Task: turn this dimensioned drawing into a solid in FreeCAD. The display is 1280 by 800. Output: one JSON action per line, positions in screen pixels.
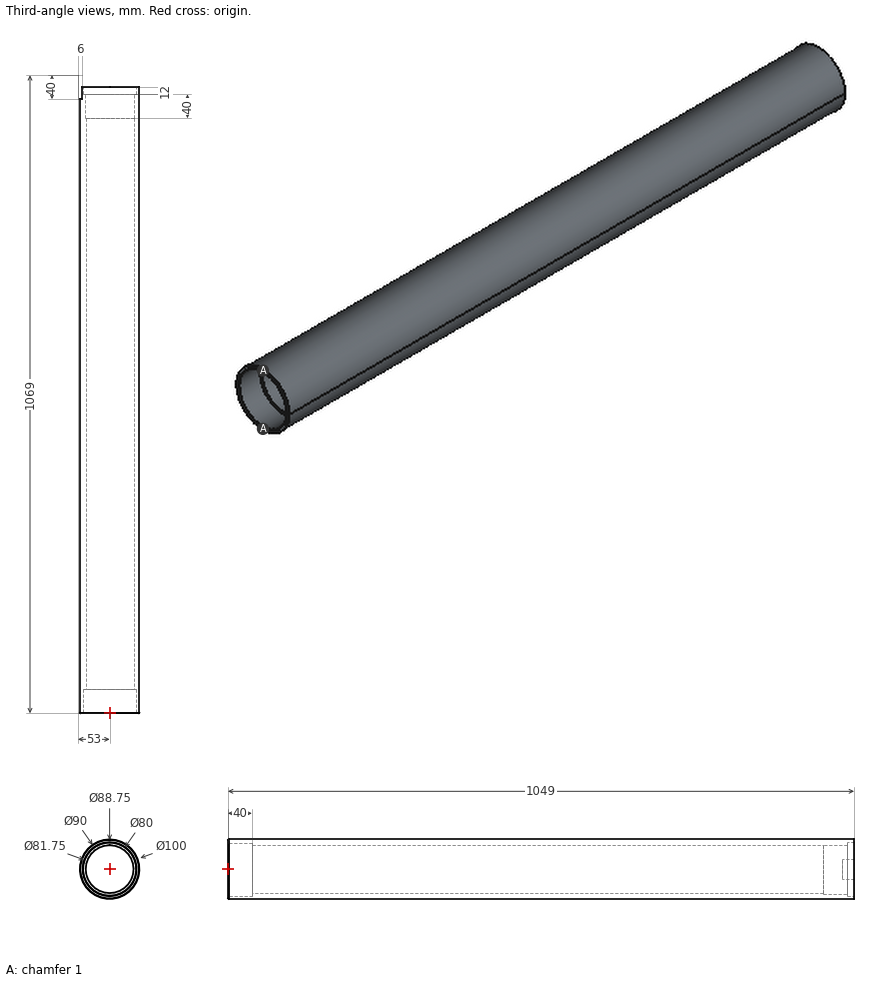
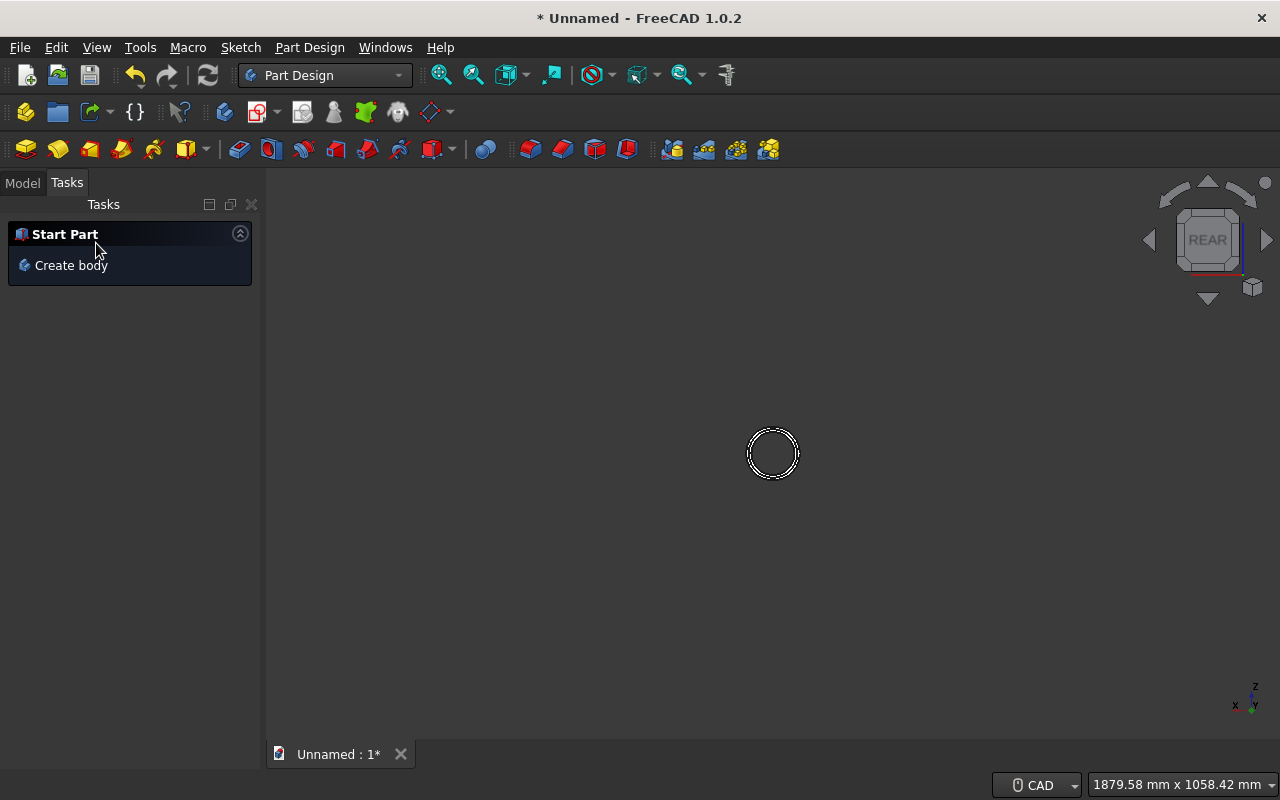
{"action": "left_click", "coordinate": [442, 76]}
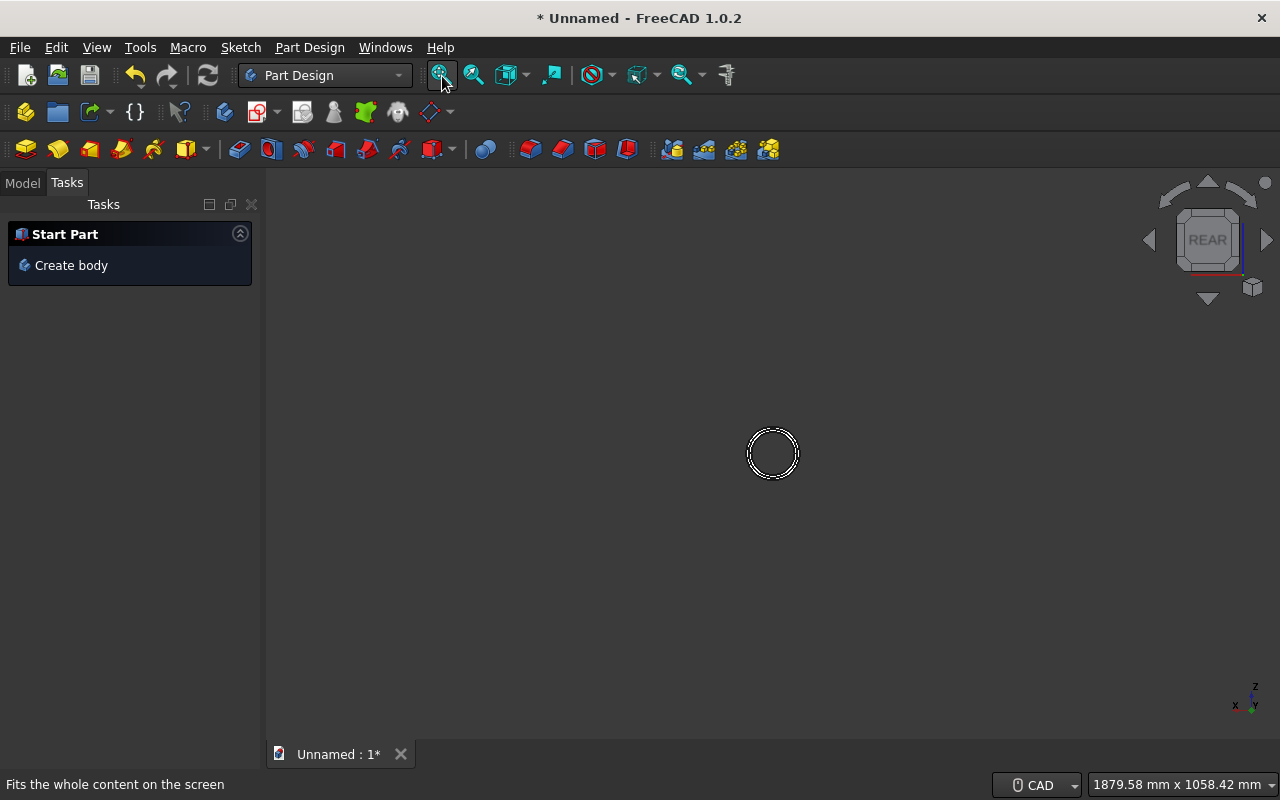
{"action": "scroll", "coordinate": [766, 432], "scroll_direction": "up", "scroll_amount": 15}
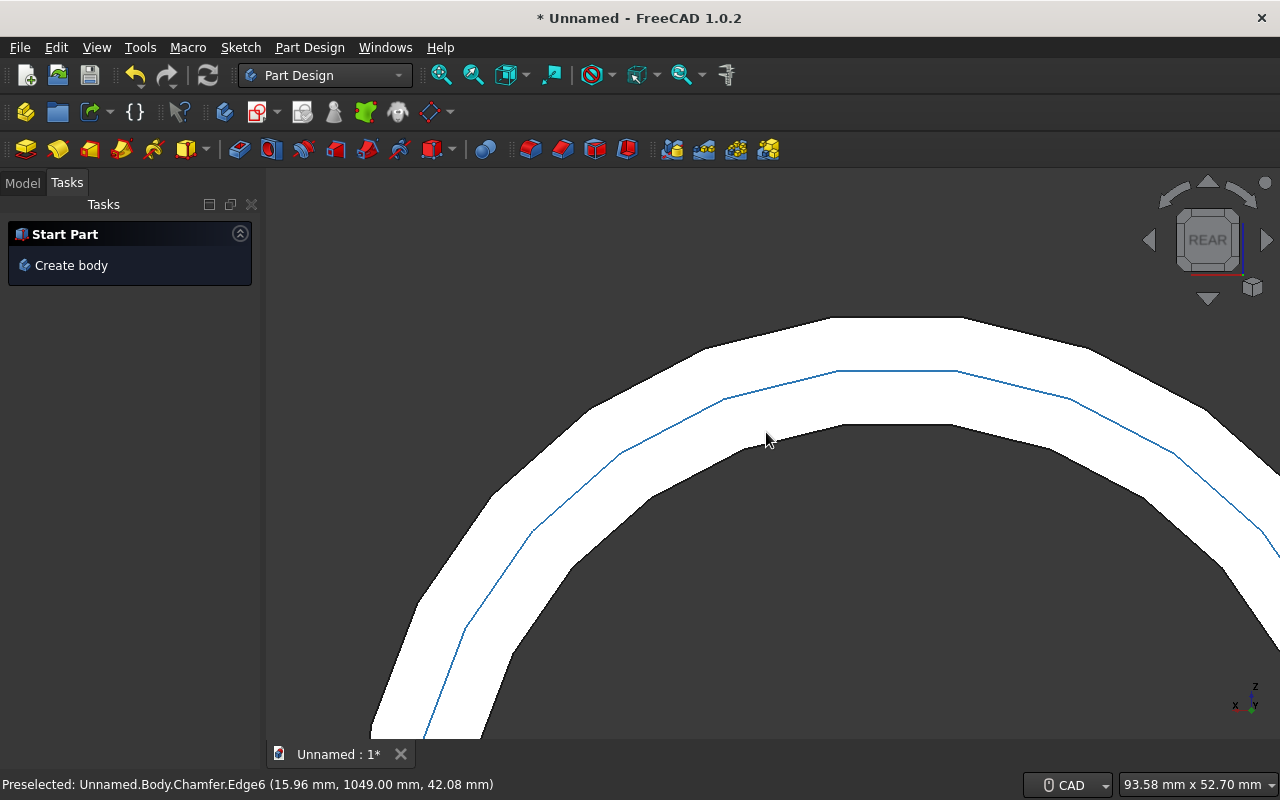
{"action": "left_click", "coordinate": [758, 436]}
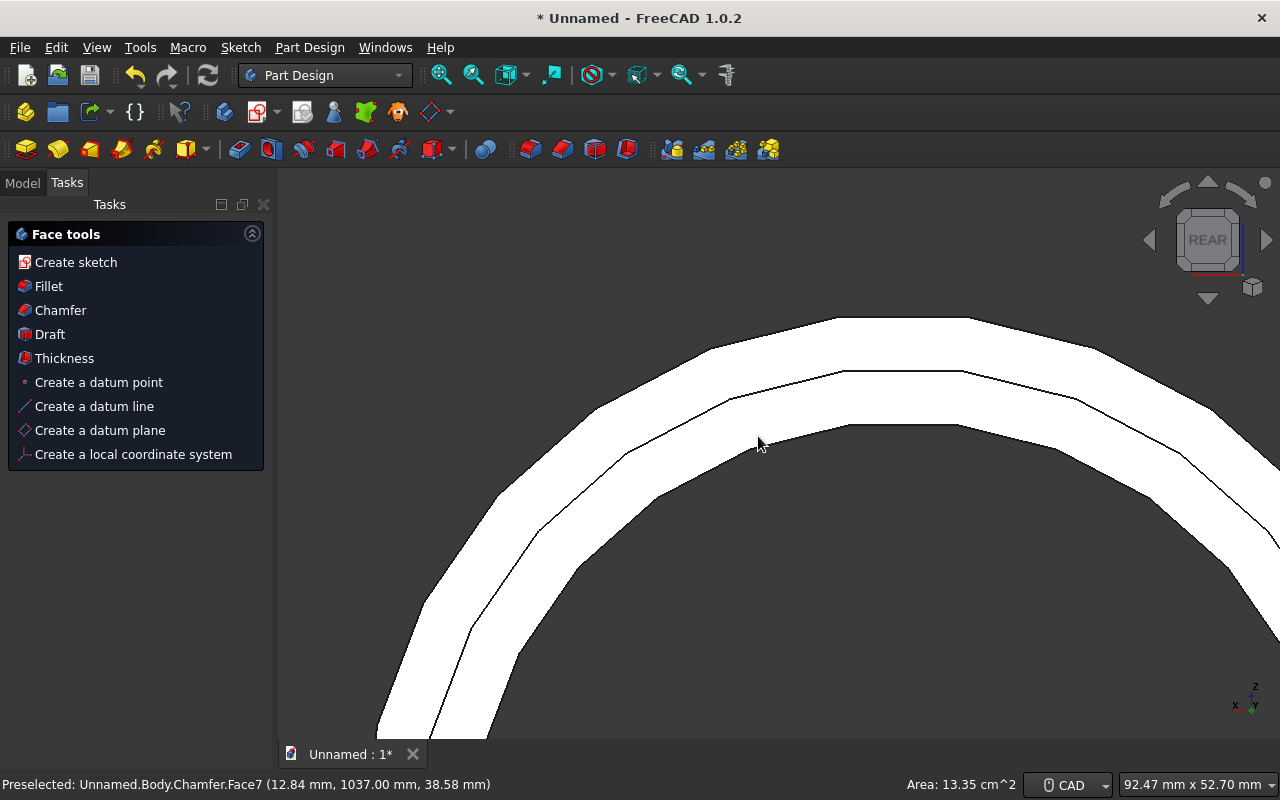
{"action": "left_click", "coordinate": [258, 112]}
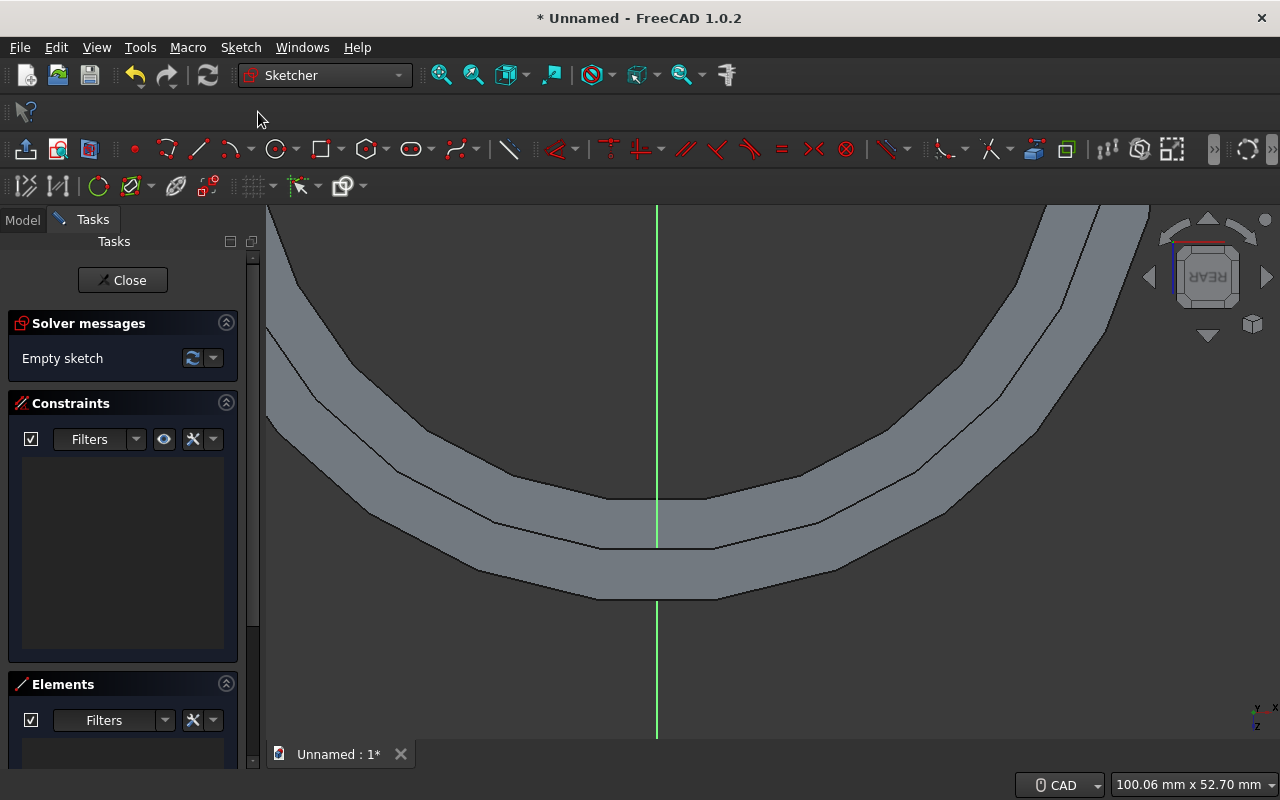
{"action": "left_click", "coordinate": [90, 150]}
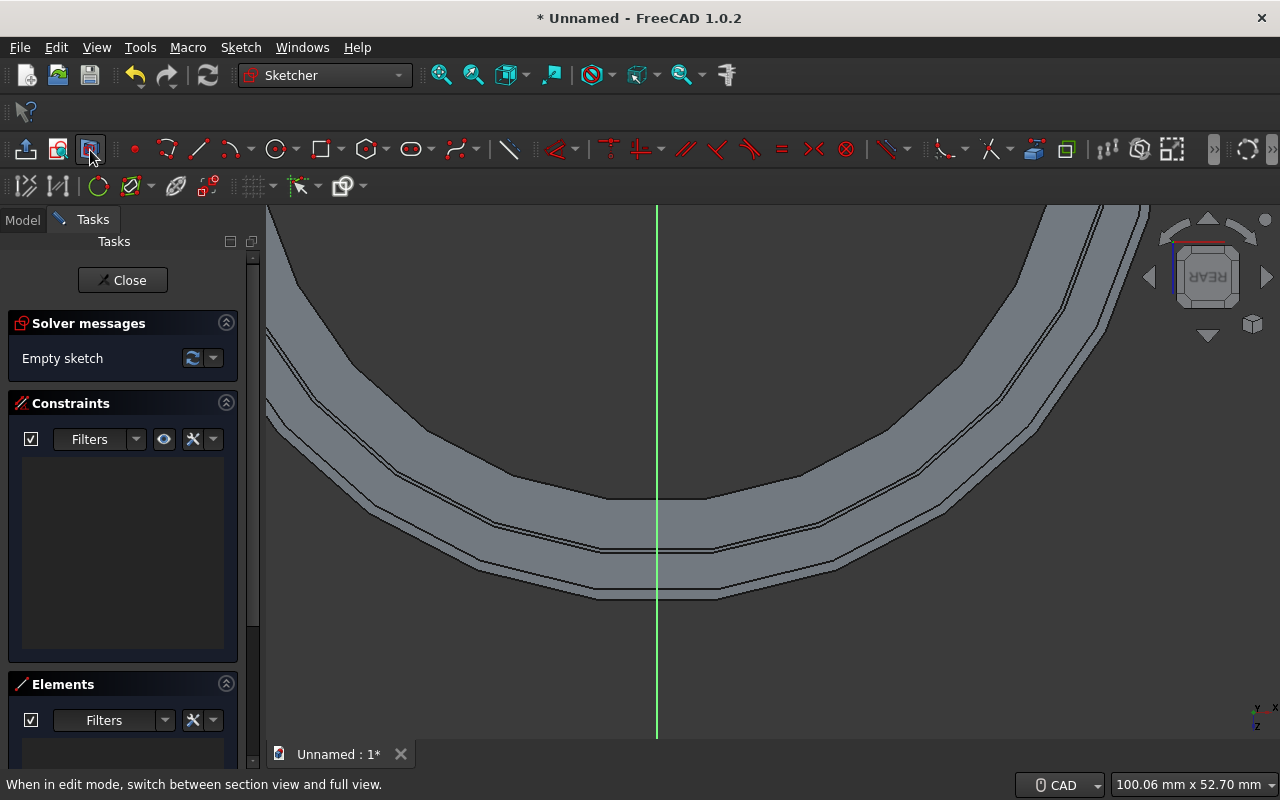
{"action": "scroll", "coordinate": [732, 691], "scroll_direction": "down", "scroll_amount": 5}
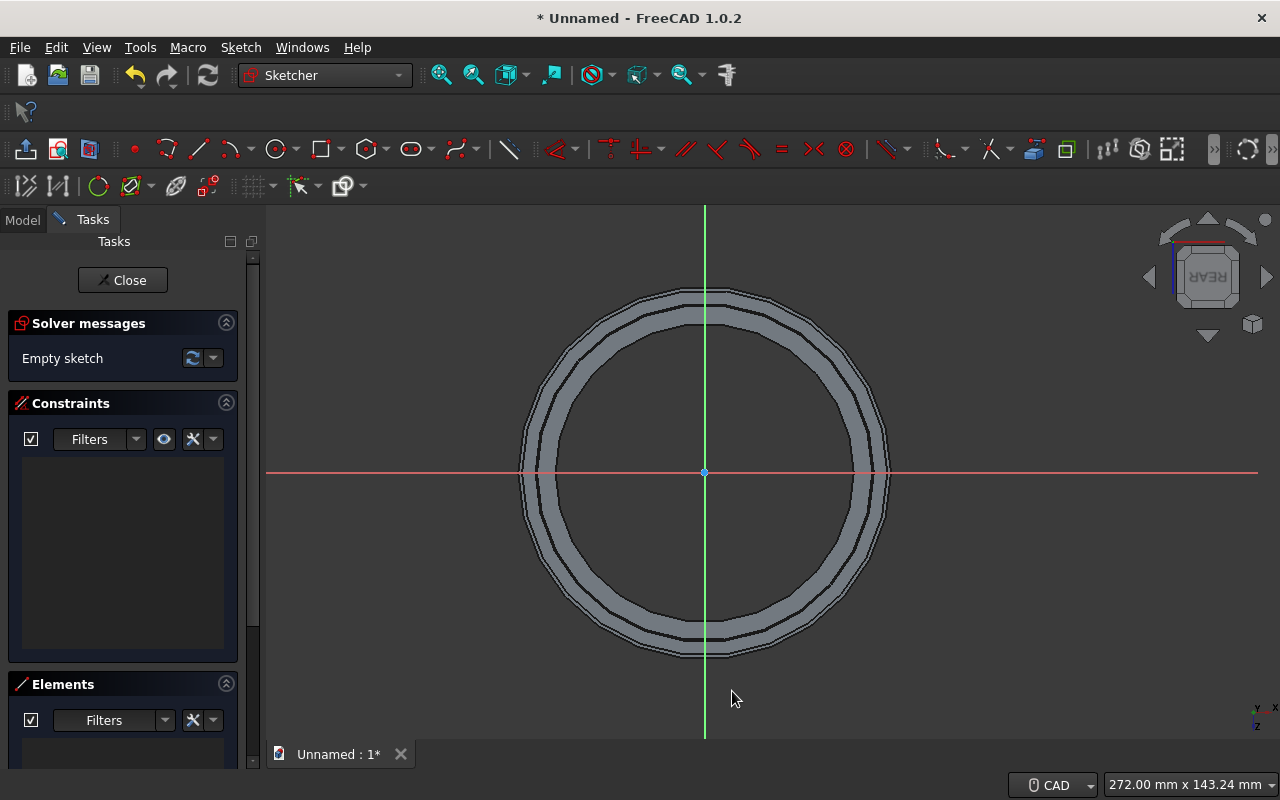
{"action": "left_click", "coordinate": [276, 150]}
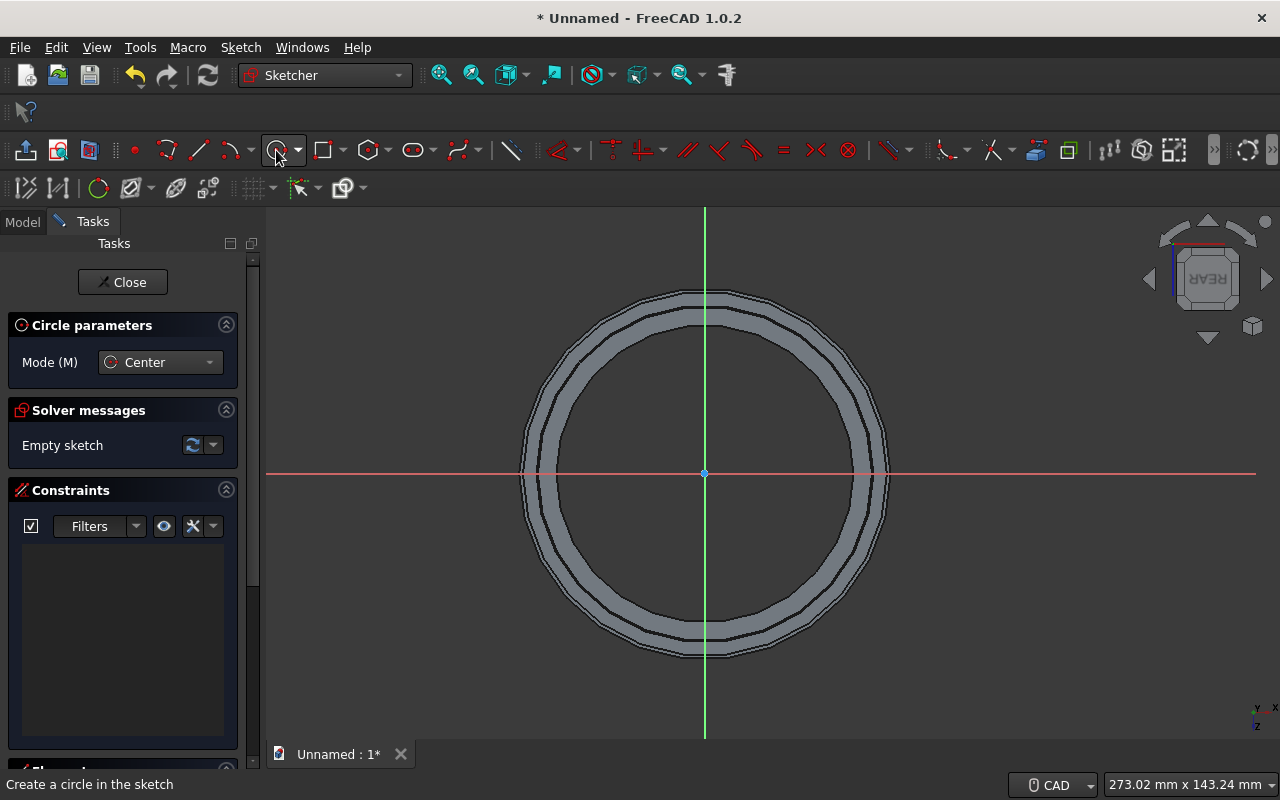
{"action": "left_click", "coordinate": [705, 474]}
{"action": "mouse_move", "coordinate": [812, 367]}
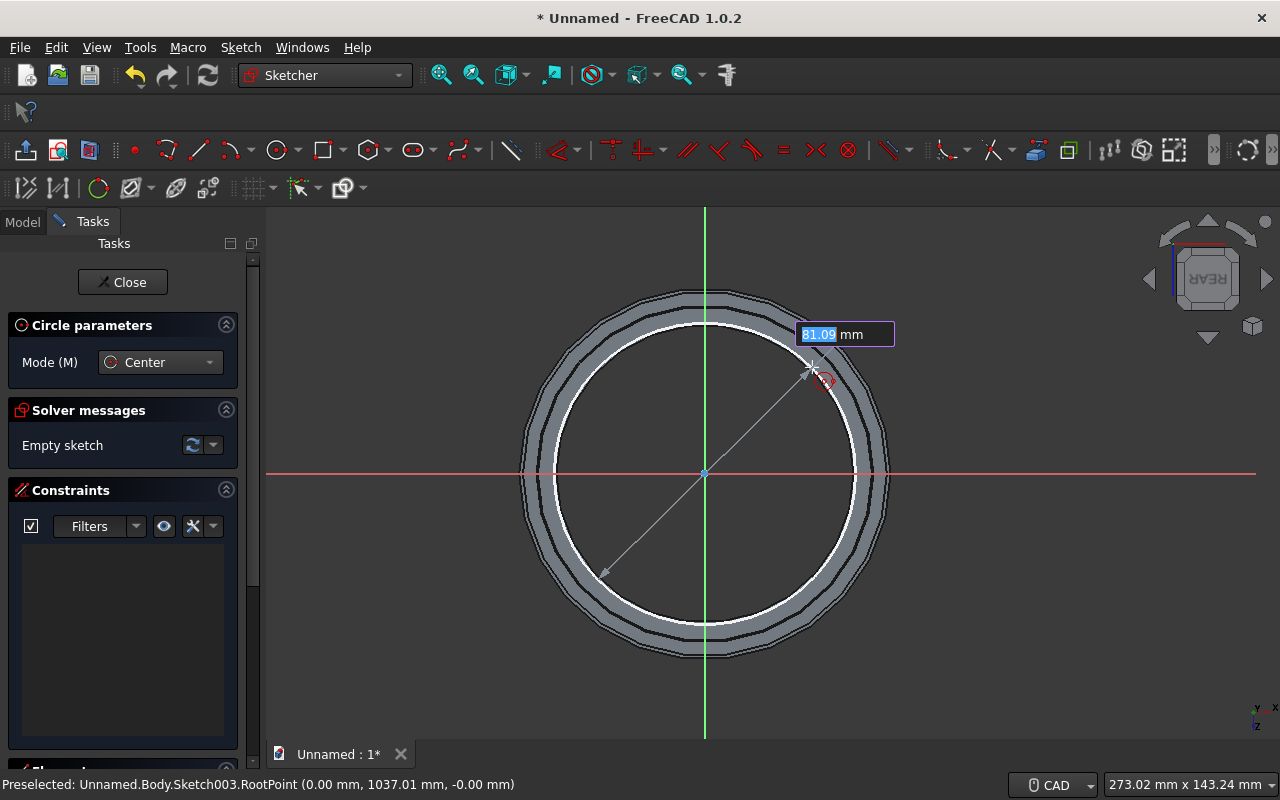
{"action": "type", "text": "81.75"}
{"action": "key", "text": "Return"}
{"action": "key", "text": "Escape"}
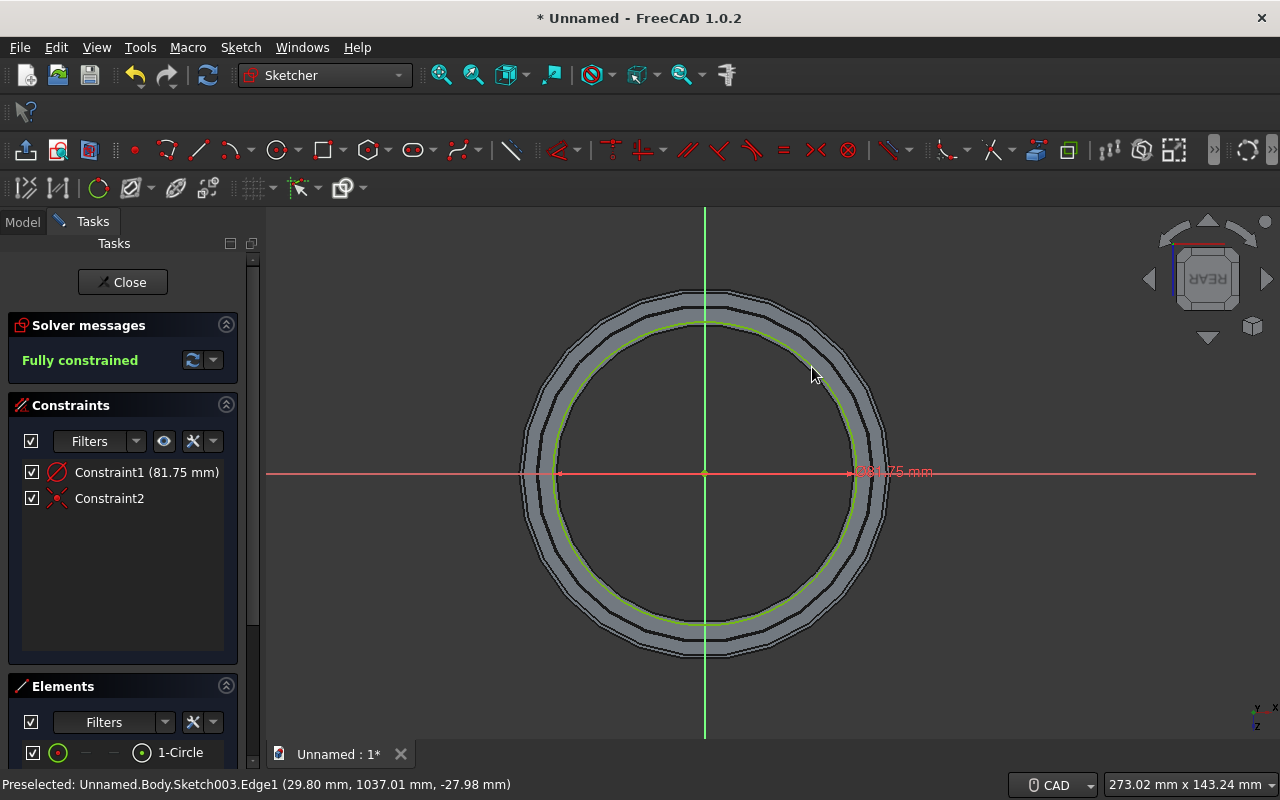
{"action": "left_click", "coordinate": [123, 282]}